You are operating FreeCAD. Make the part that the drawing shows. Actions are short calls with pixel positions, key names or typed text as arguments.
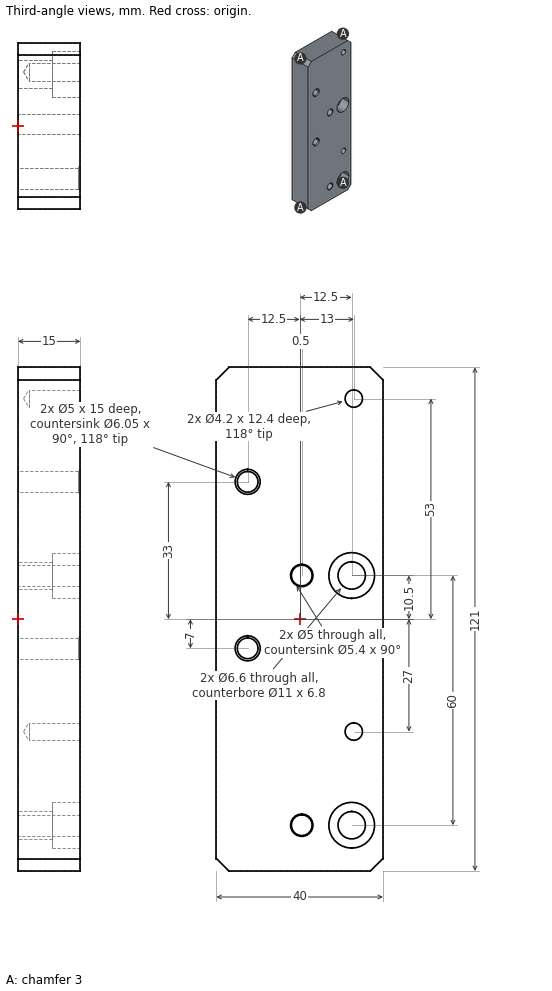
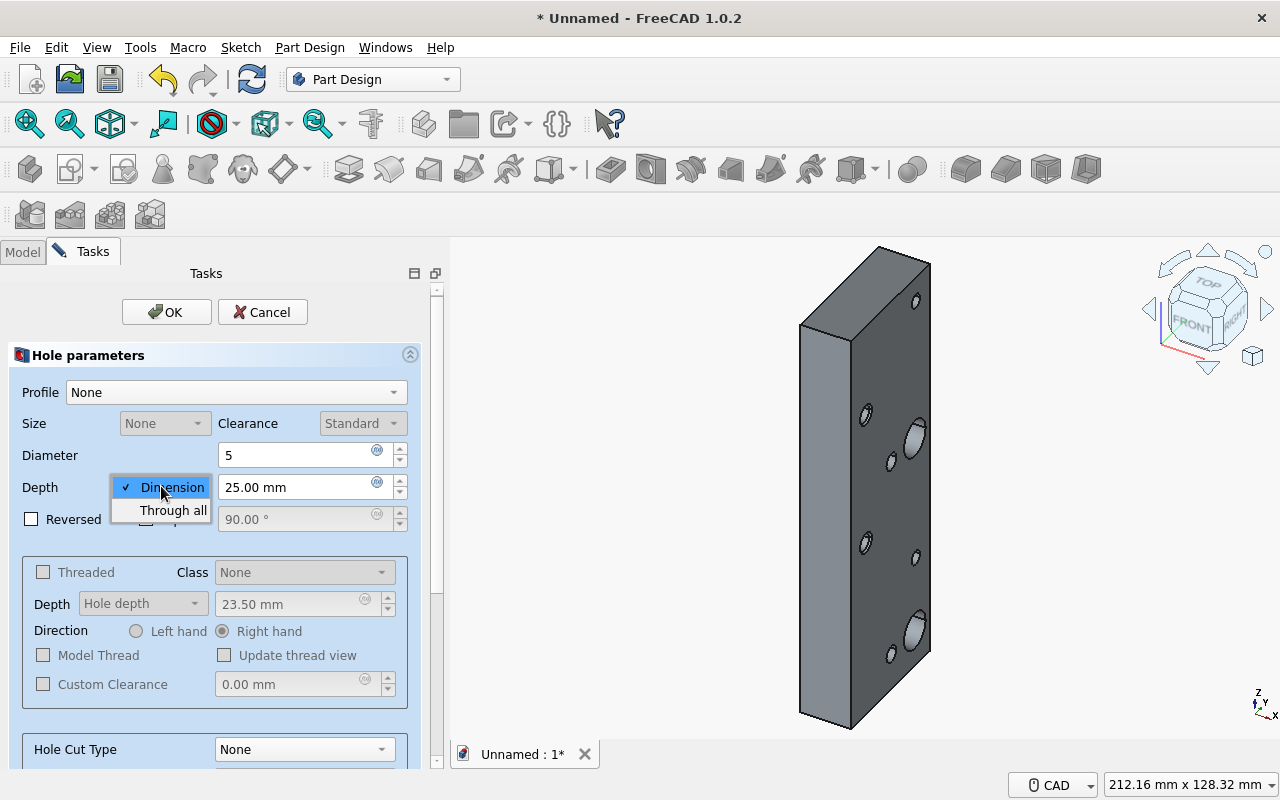
click(160, 510)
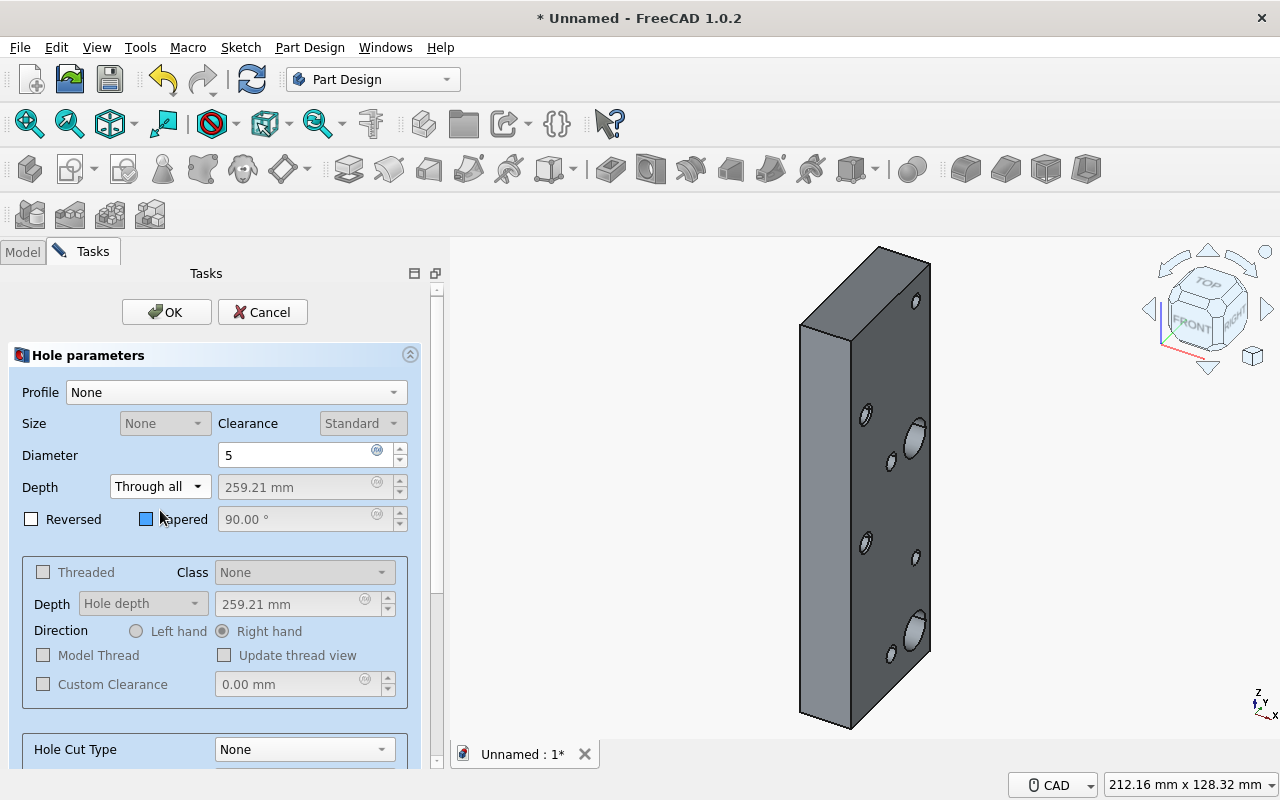
click(306, 750)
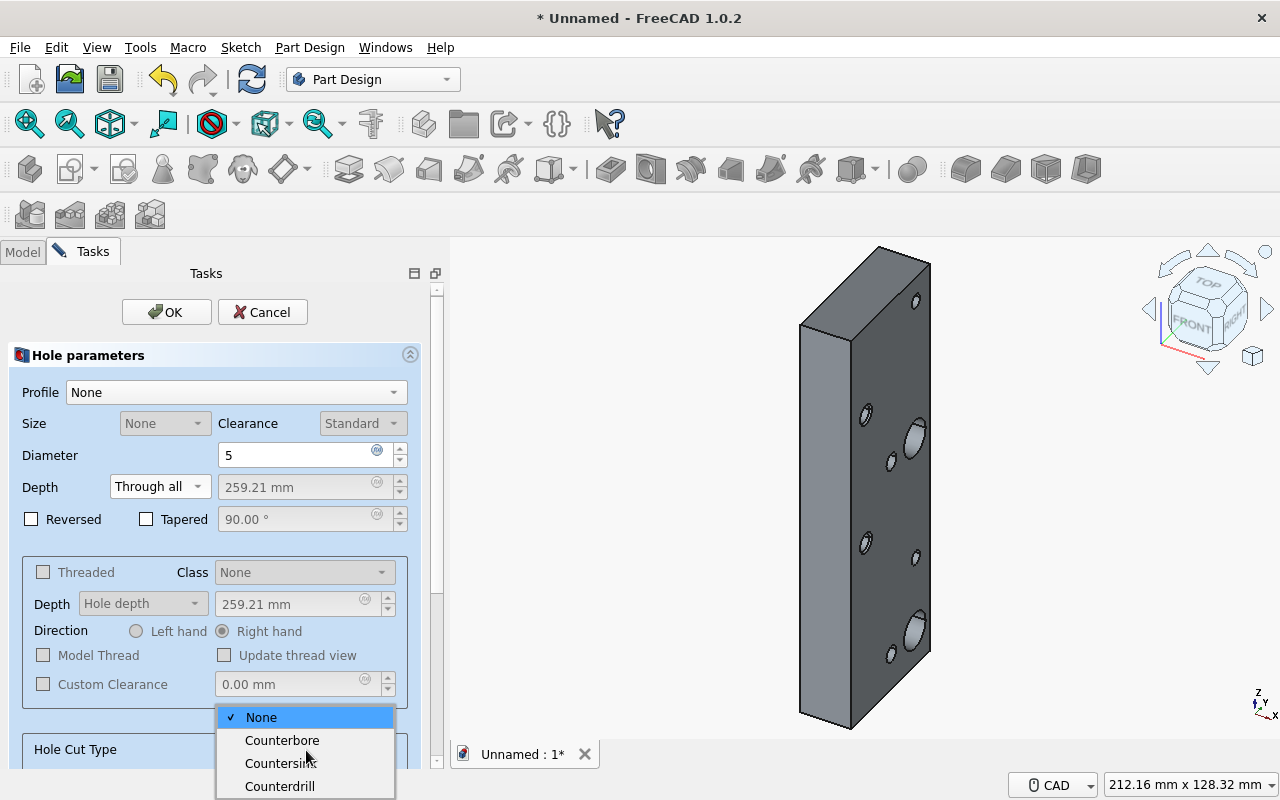
click(304, 764)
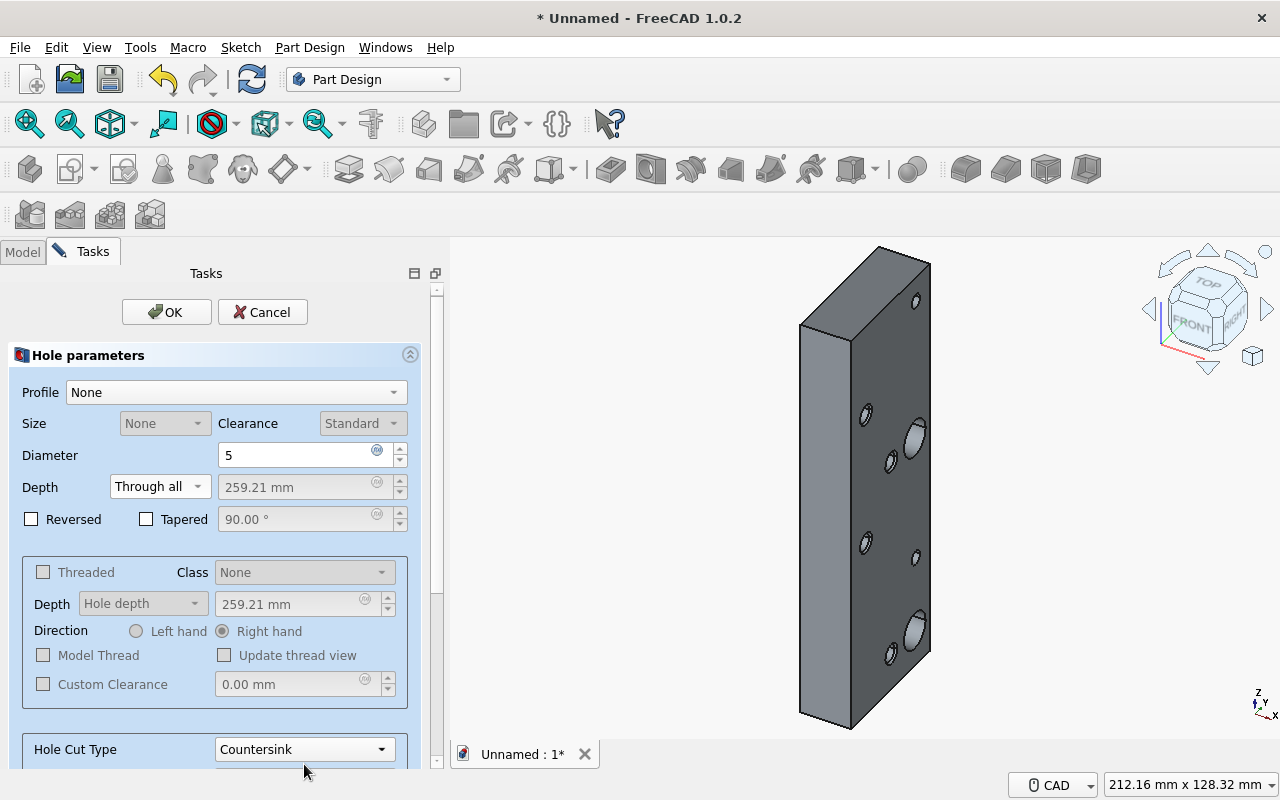
scroll(437, 526, down, 2)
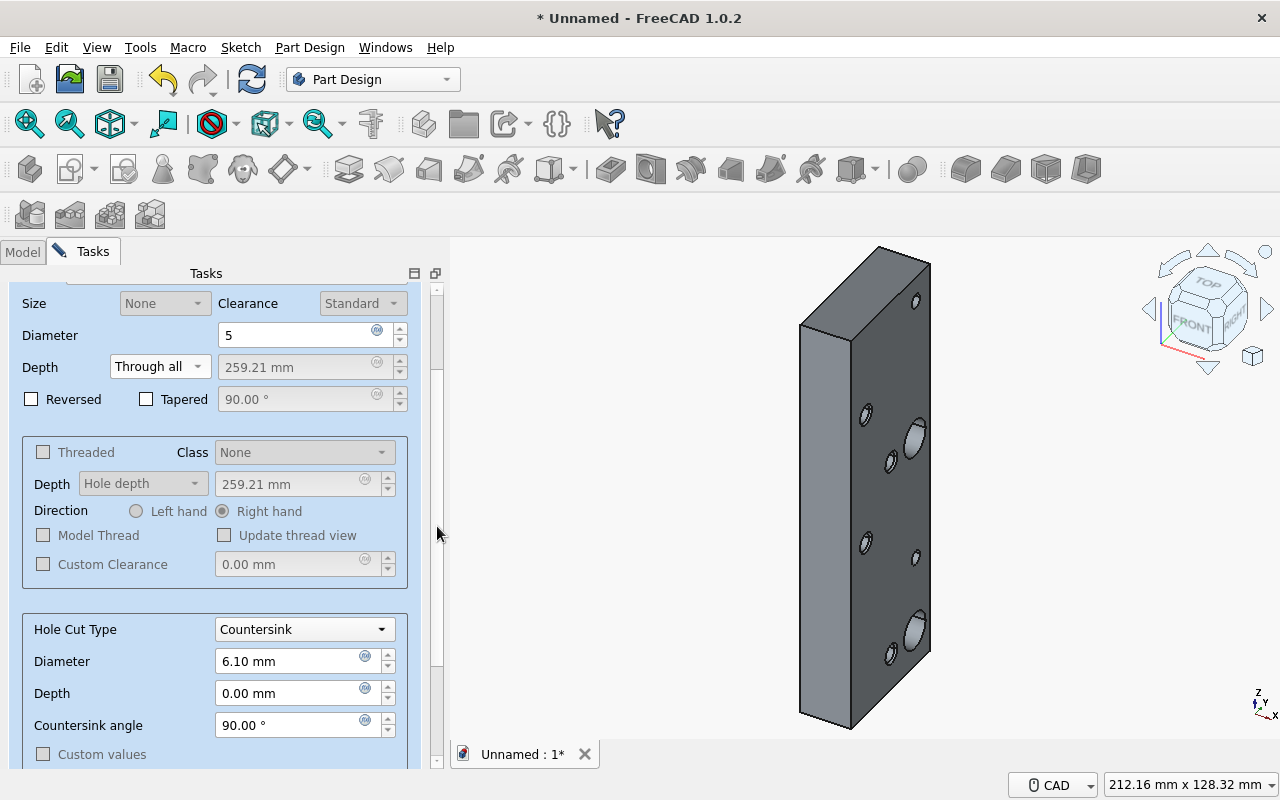
triple_click(298, 661)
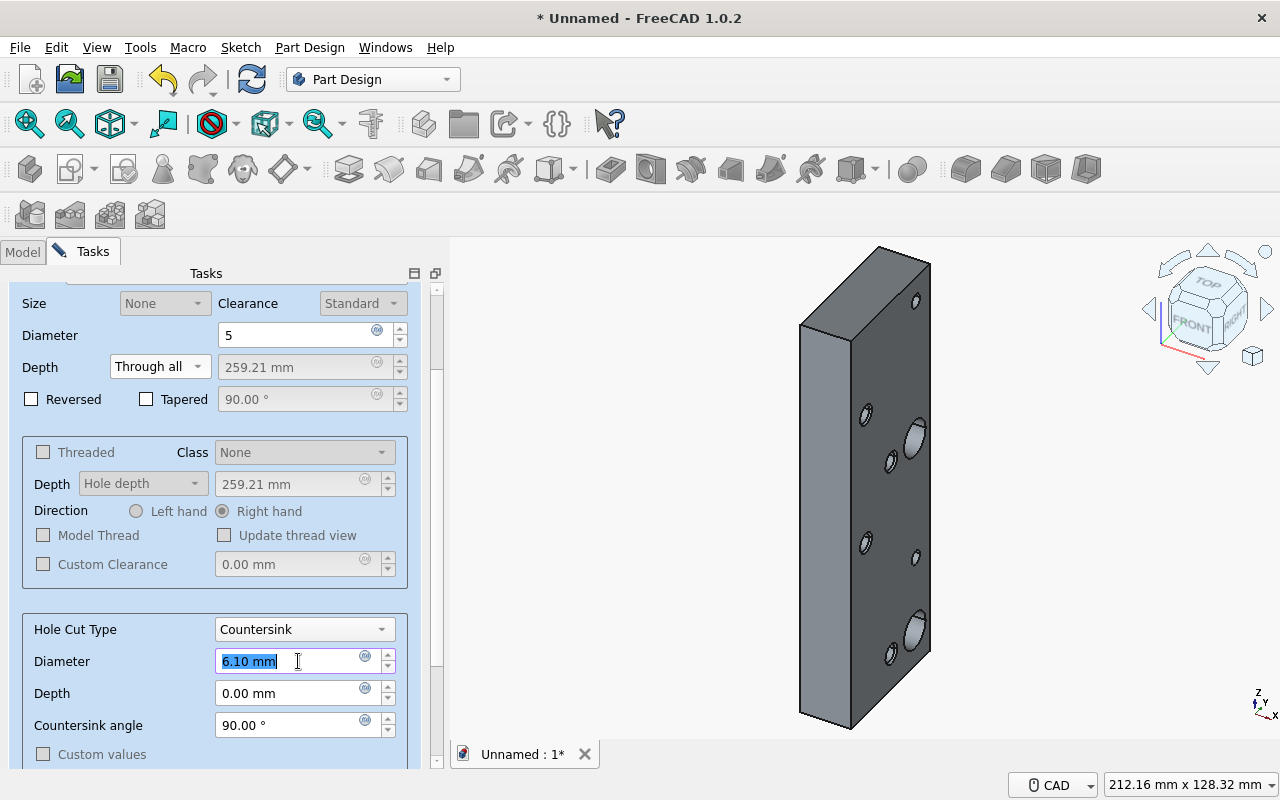
text(5.4)
key(Tab)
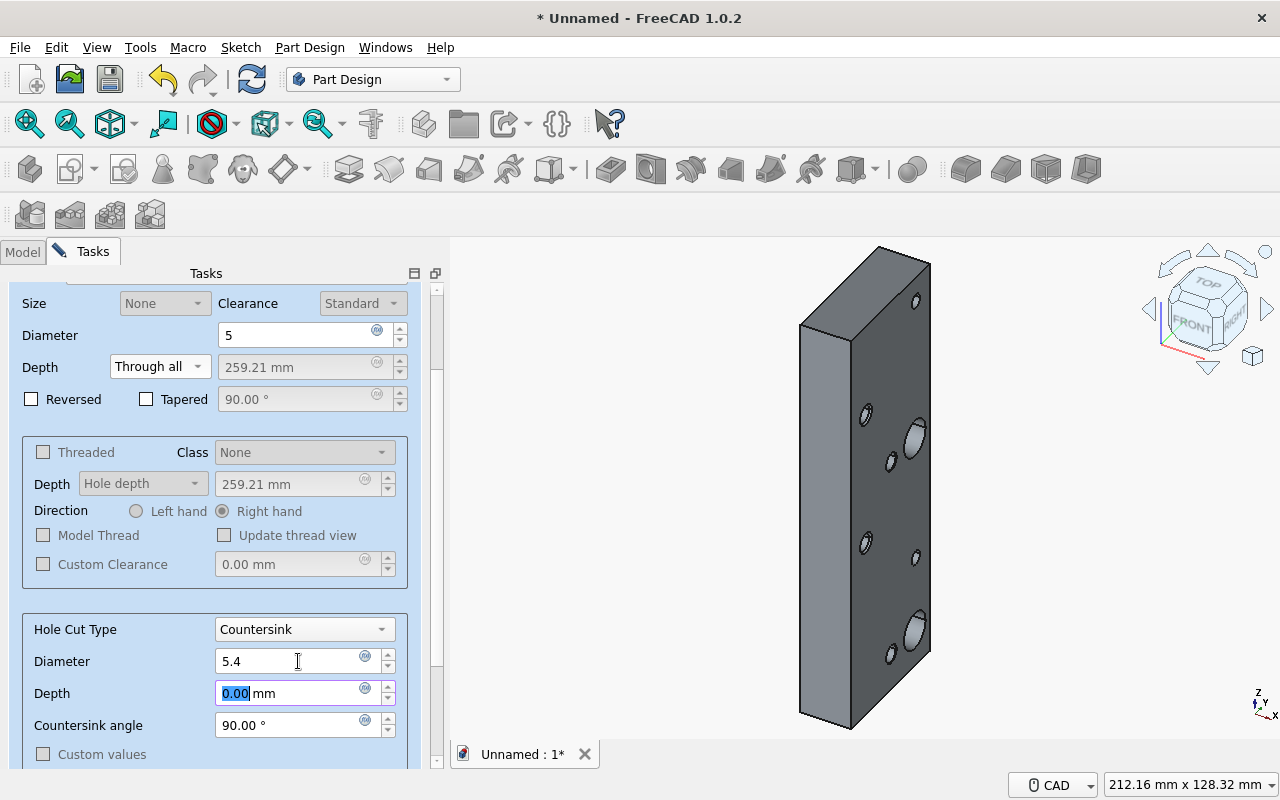
scroll(437, 526, up, 3)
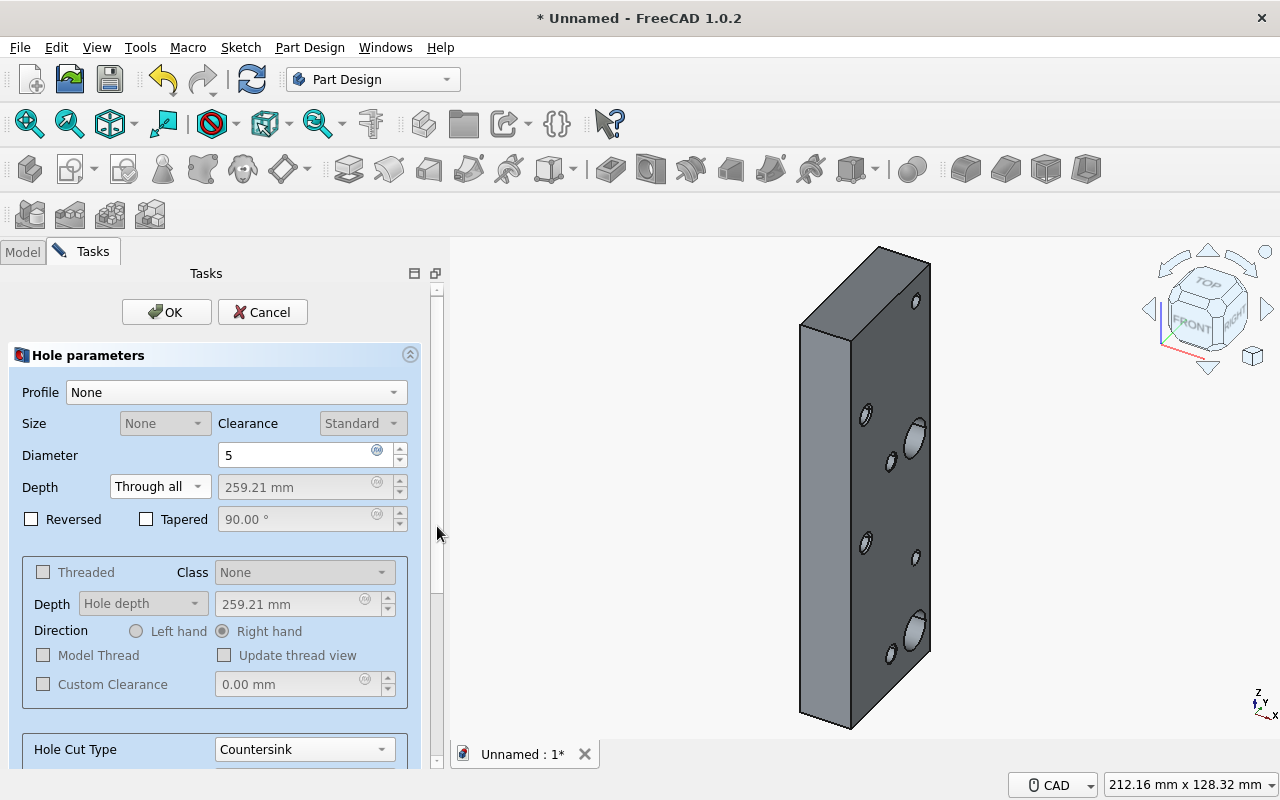
click(167, 312)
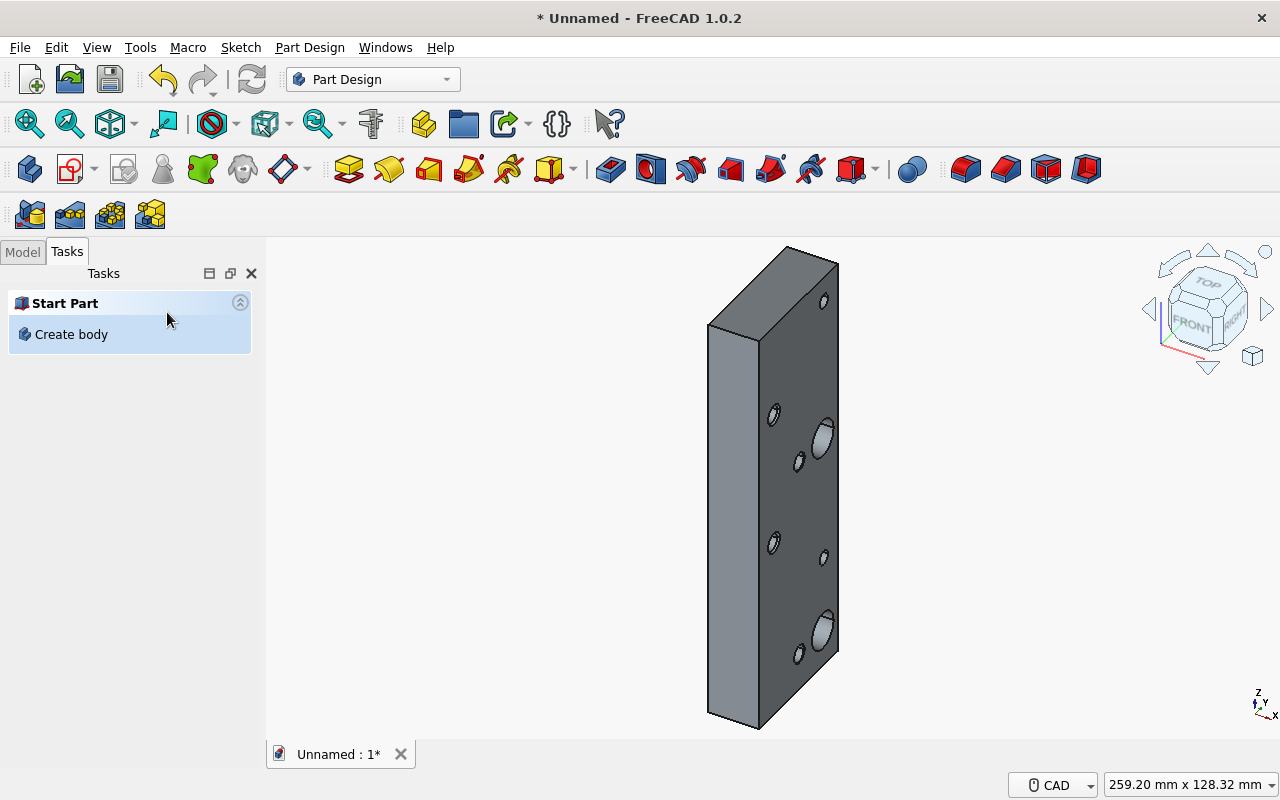
click(734, 332)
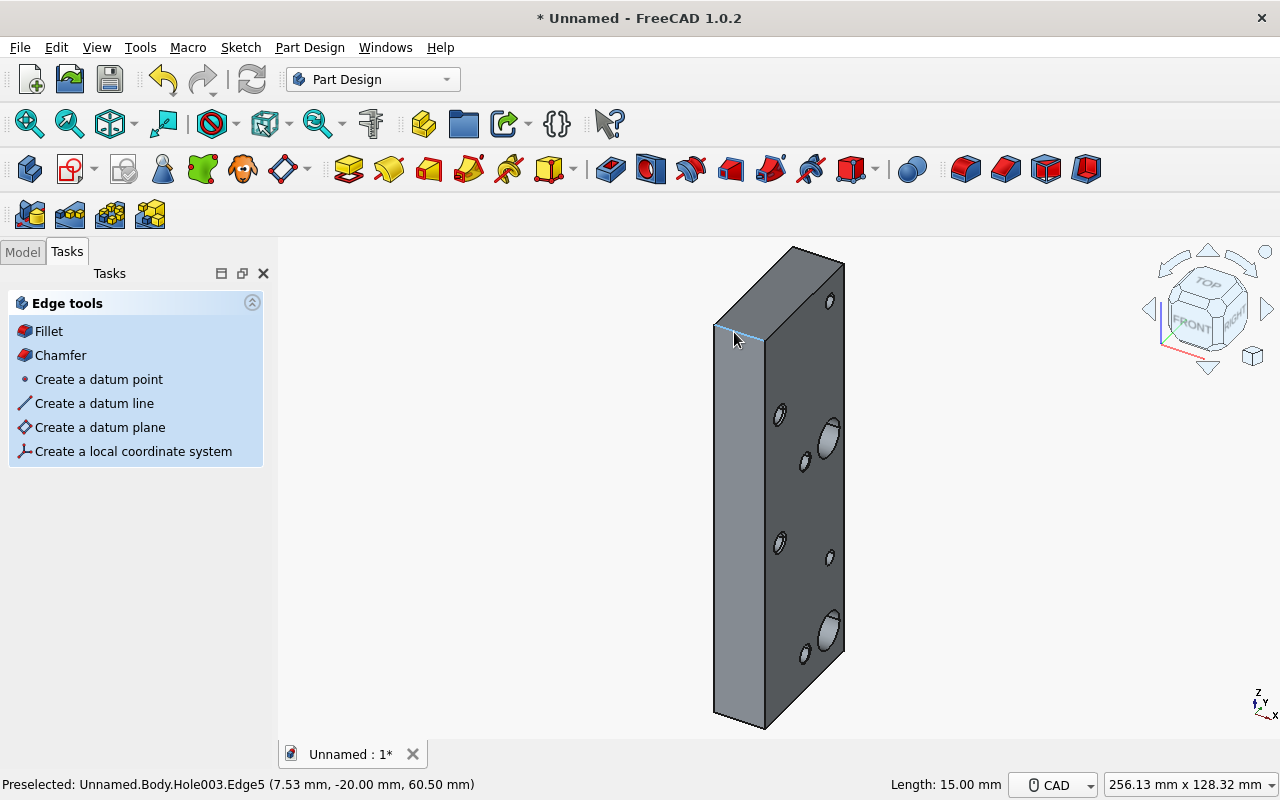
key(0)